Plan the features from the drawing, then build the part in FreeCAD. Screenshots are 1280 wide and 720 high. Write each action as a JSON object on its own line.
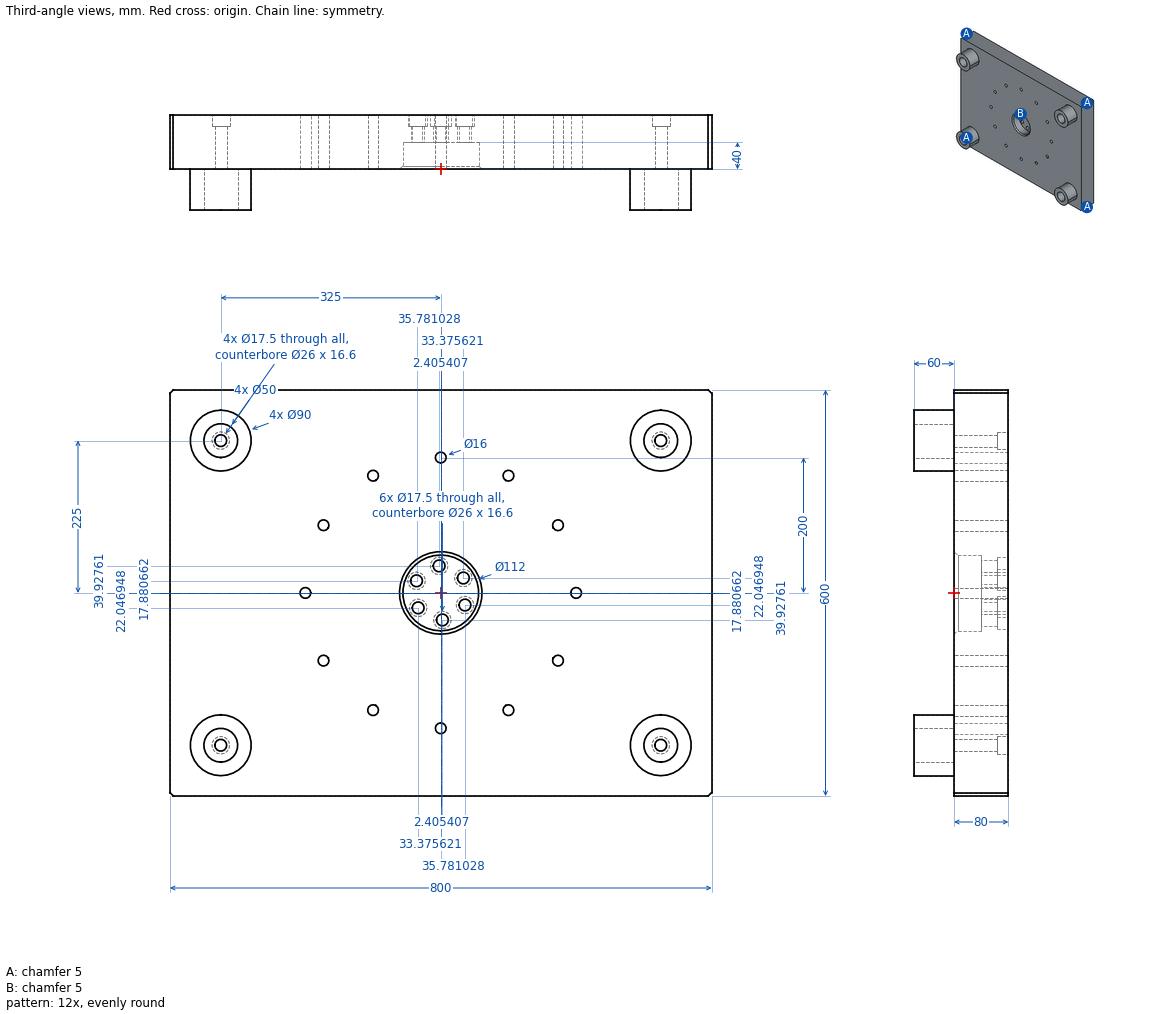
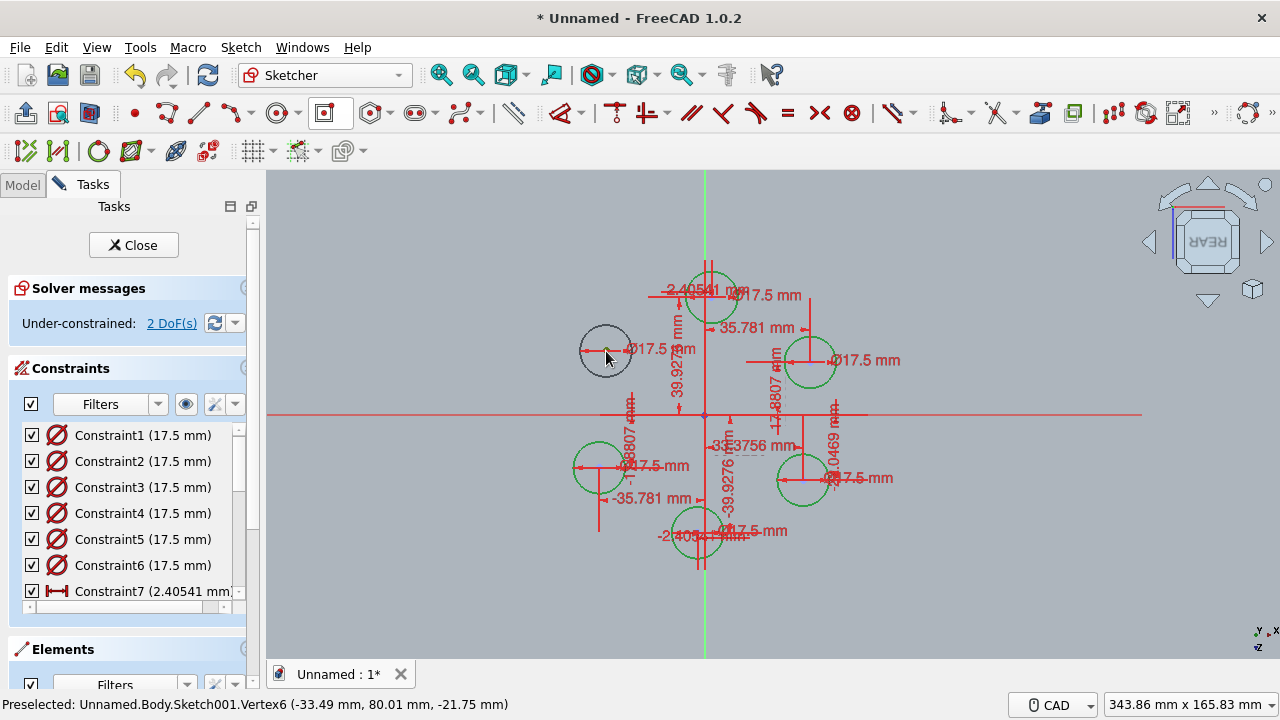
{"action": "key", "text": "l"}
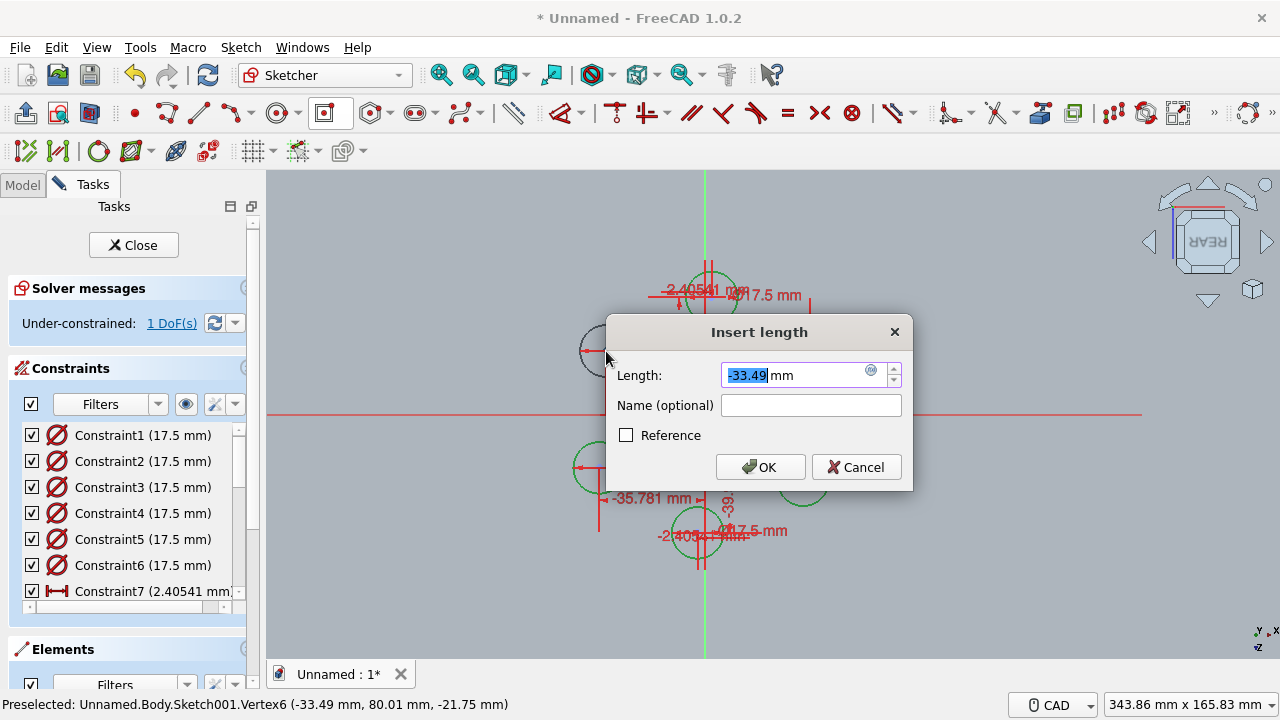
{"action": "type", "text": "-33.375621"}
{"action": "key", "text": "Return"}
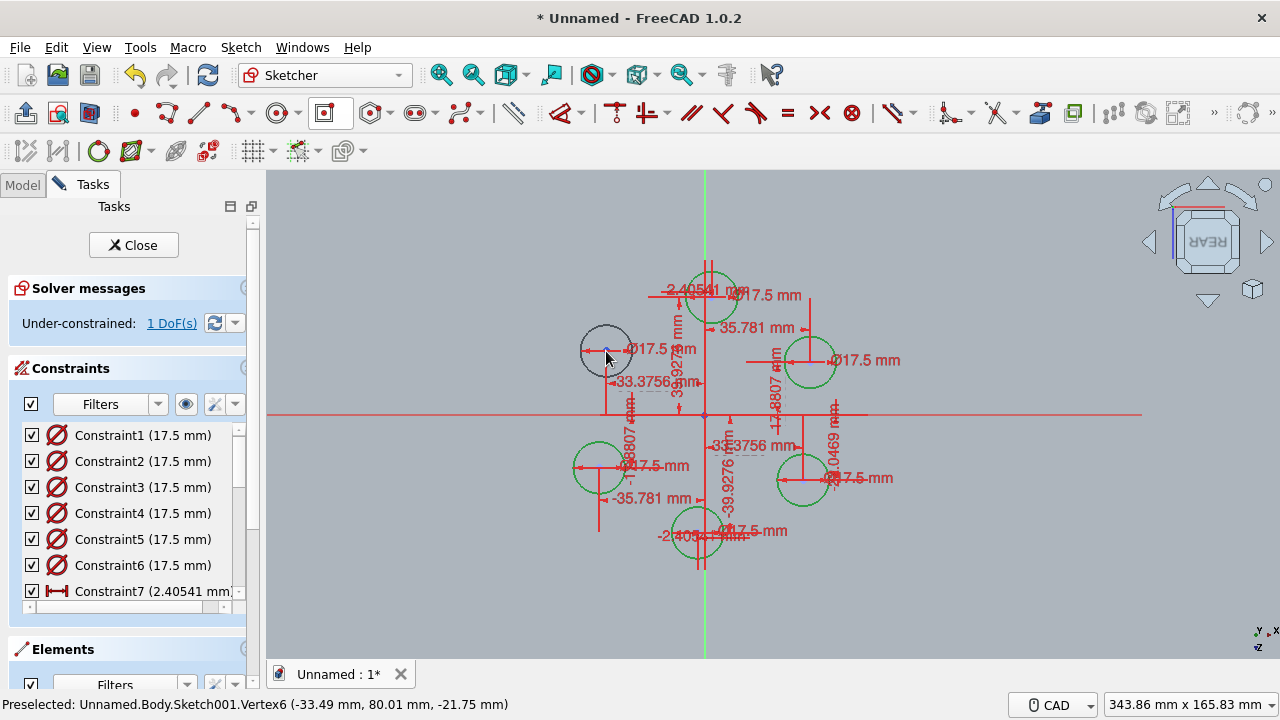
{"action": "left_click", "coordinate": [606, 351]}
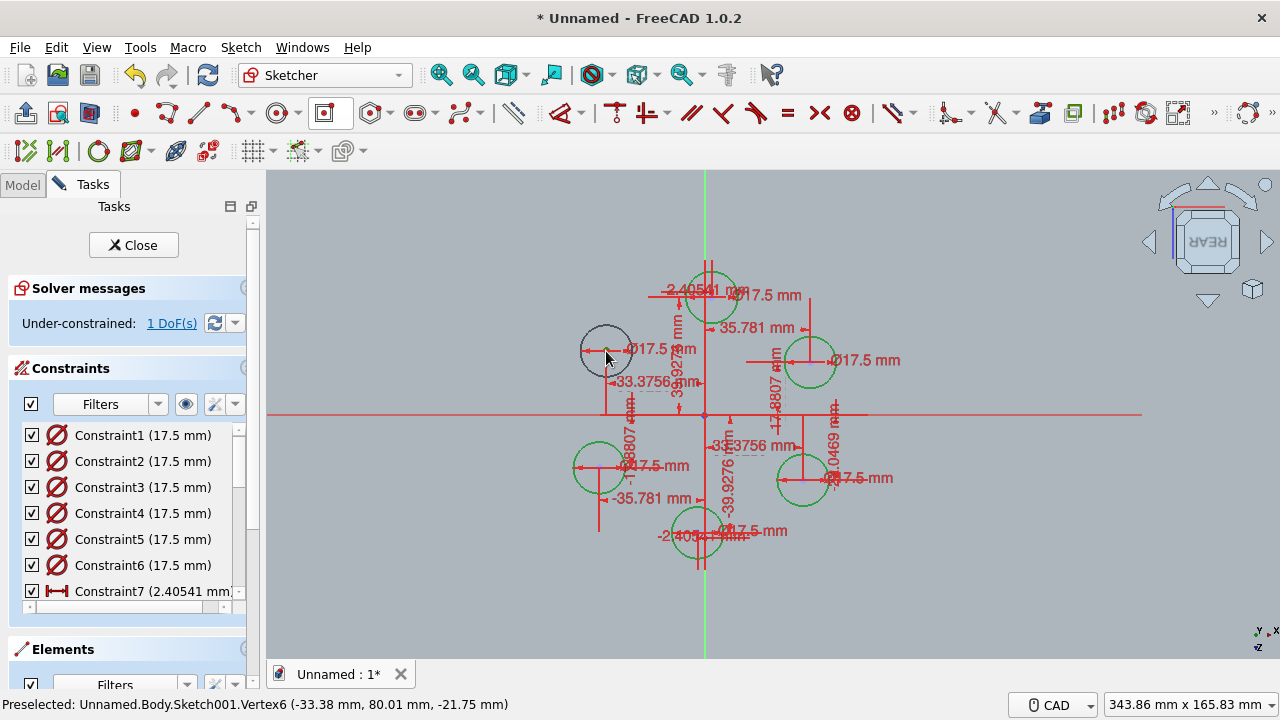
{"action": "key", "text": "i"}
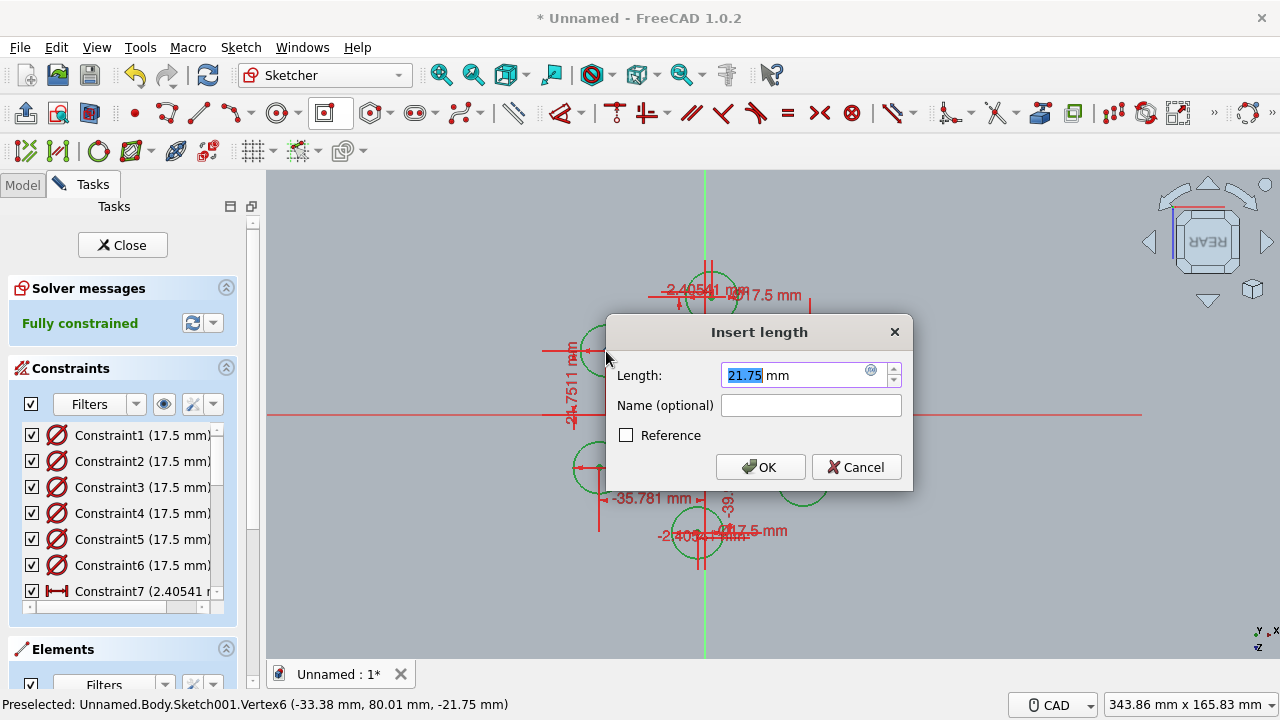
{"action": "type", "text": "22.046948"}
{"action": "key", "text": "Return"}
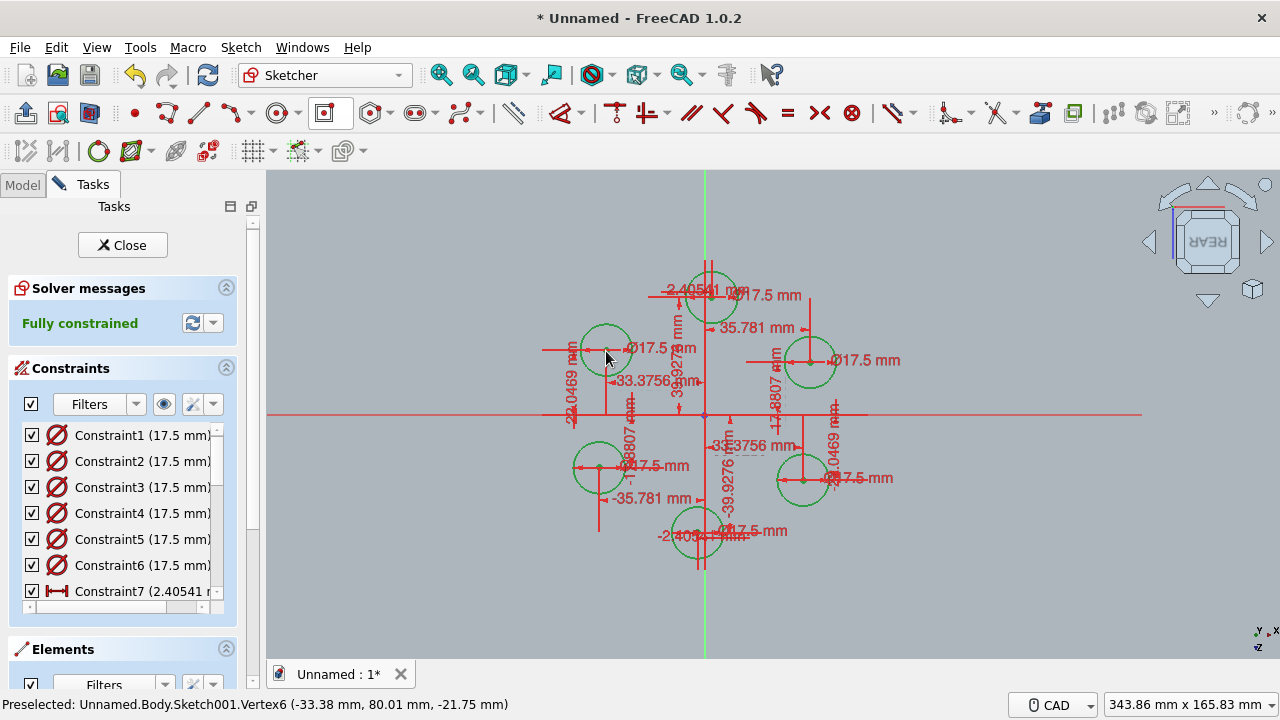
{"action": "left_click", "coordinate": [123, 245]}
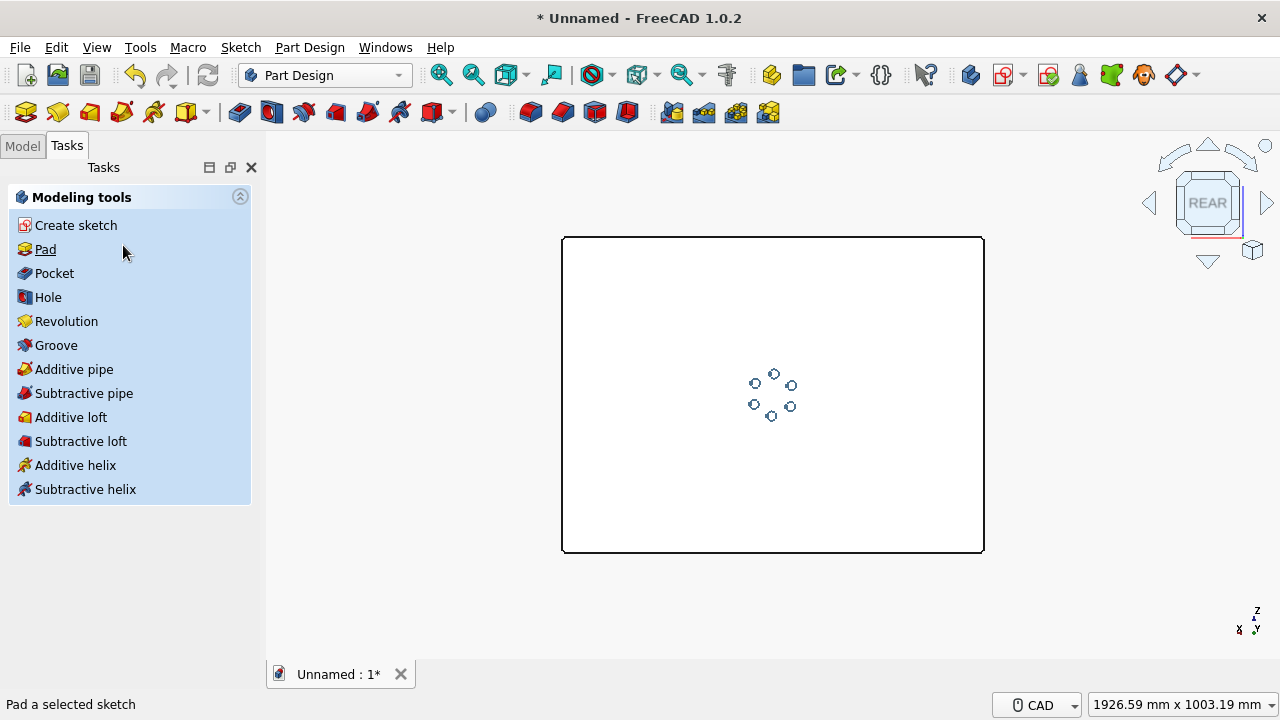
{"action": "left_click", "coordinate": [272, 112]}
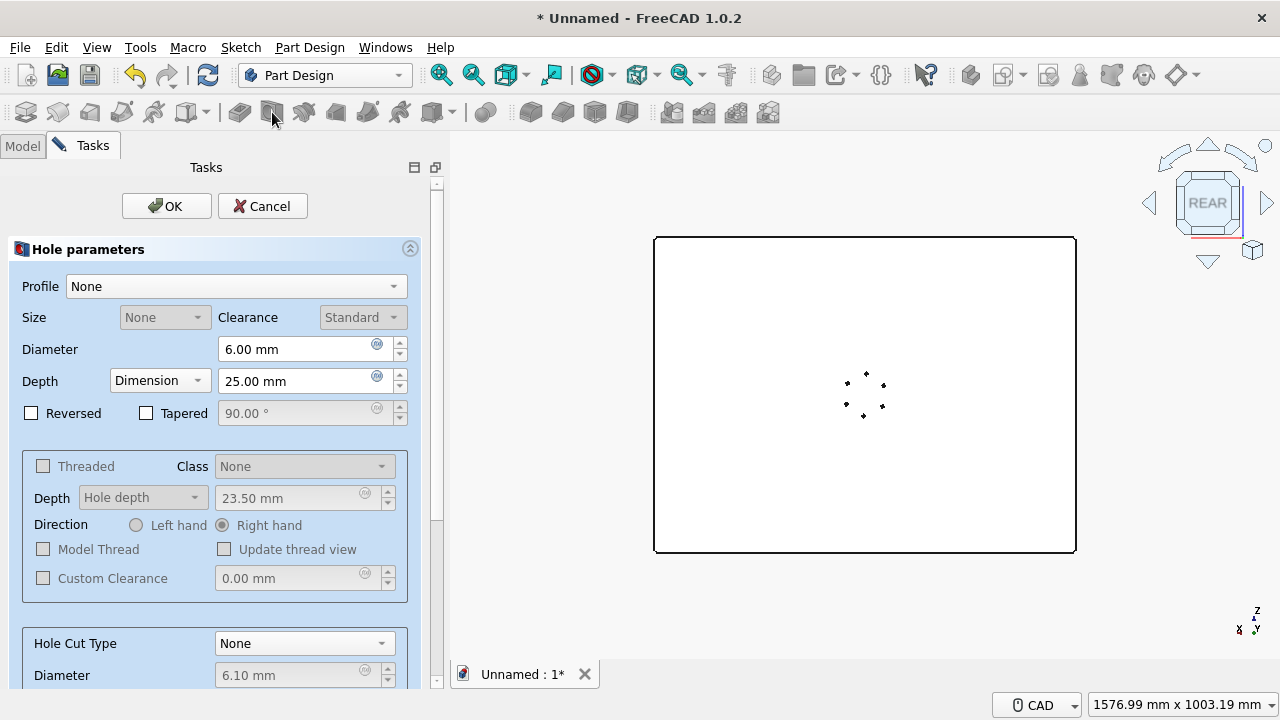
{"action": "triple_click", "coordinate": [305, 349]}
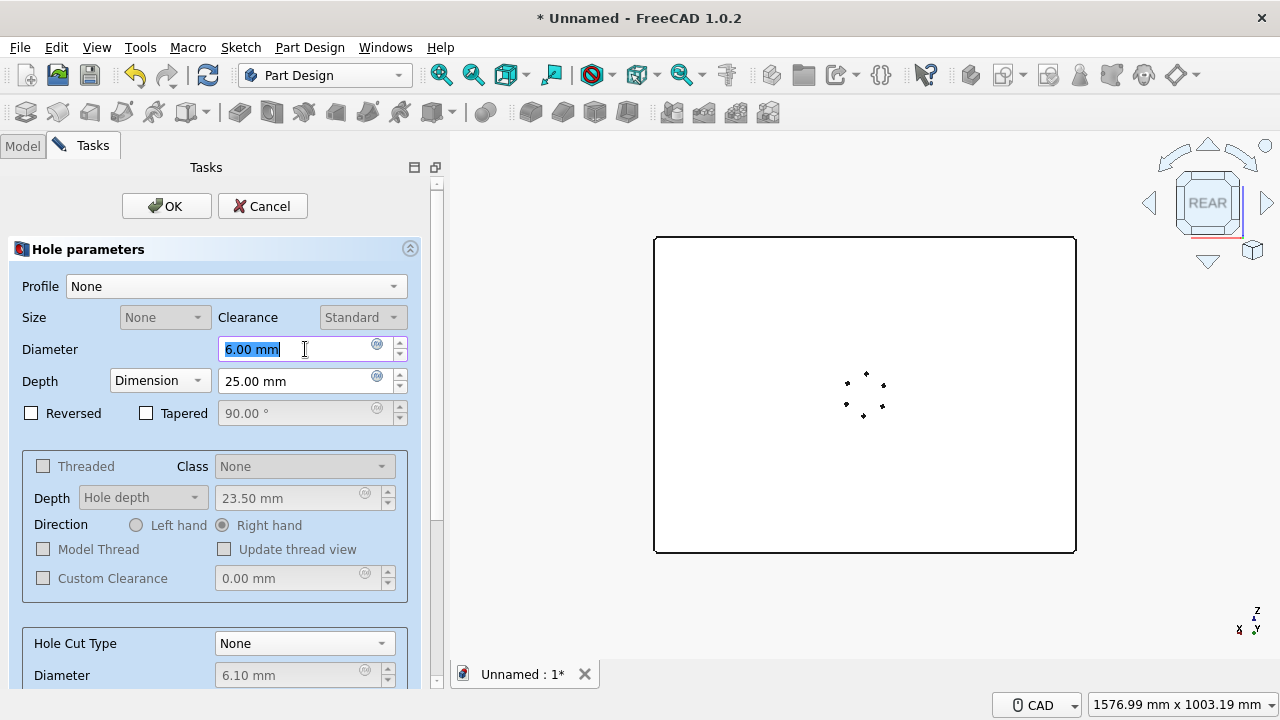
{"action": "type", "text": "17.5"}
{"action": "key", "text": "Tab"}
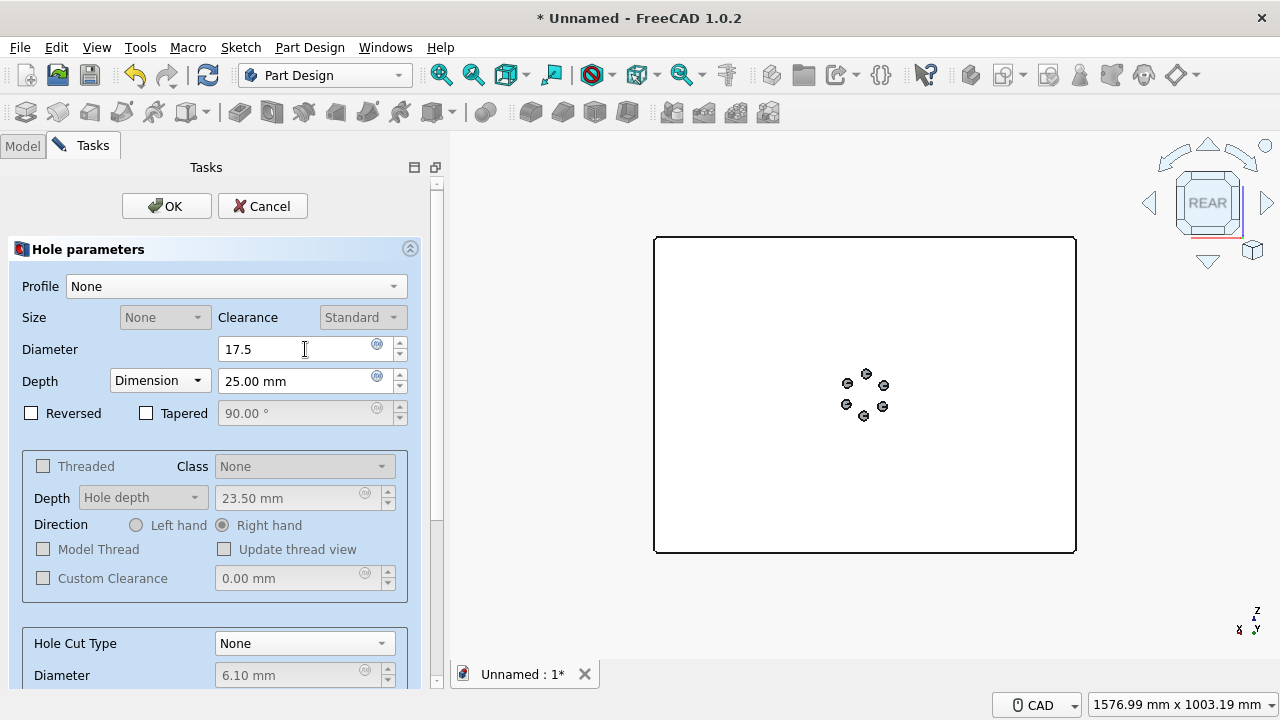
{"action": "left_click", "coordinate": [161, 380]}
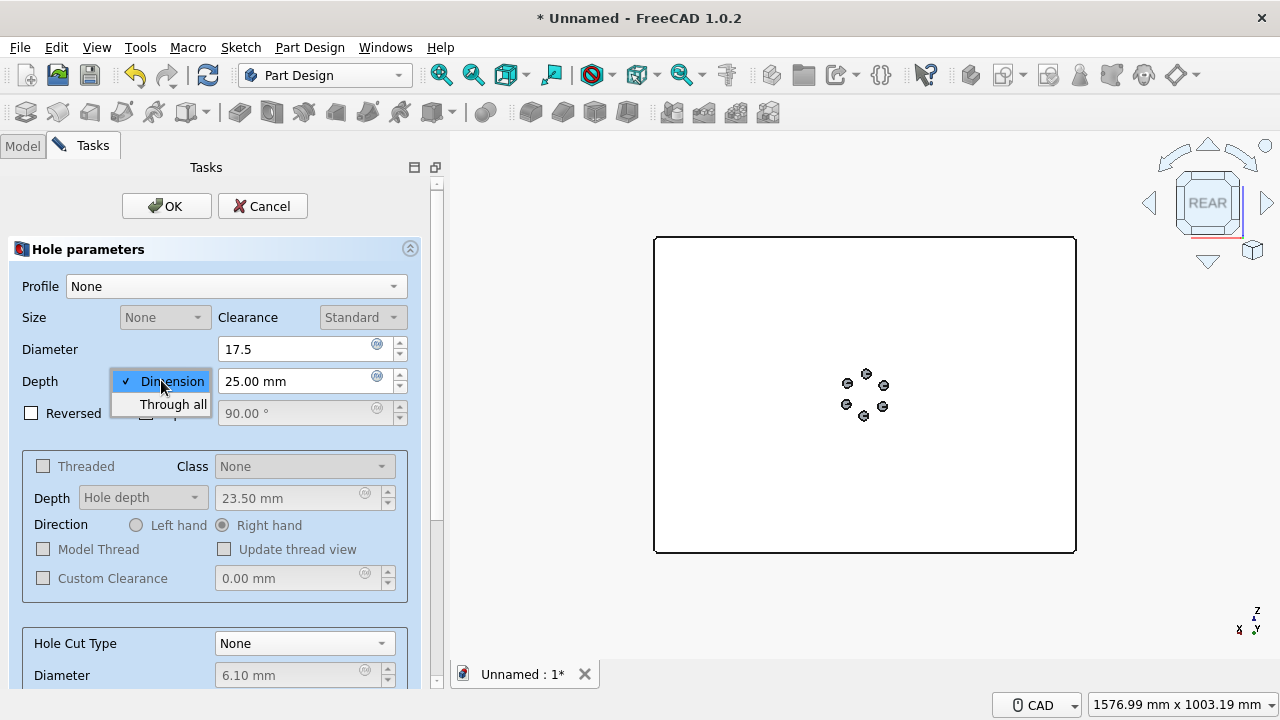
{"action": "left_click", "coordinate": [160, 404]}